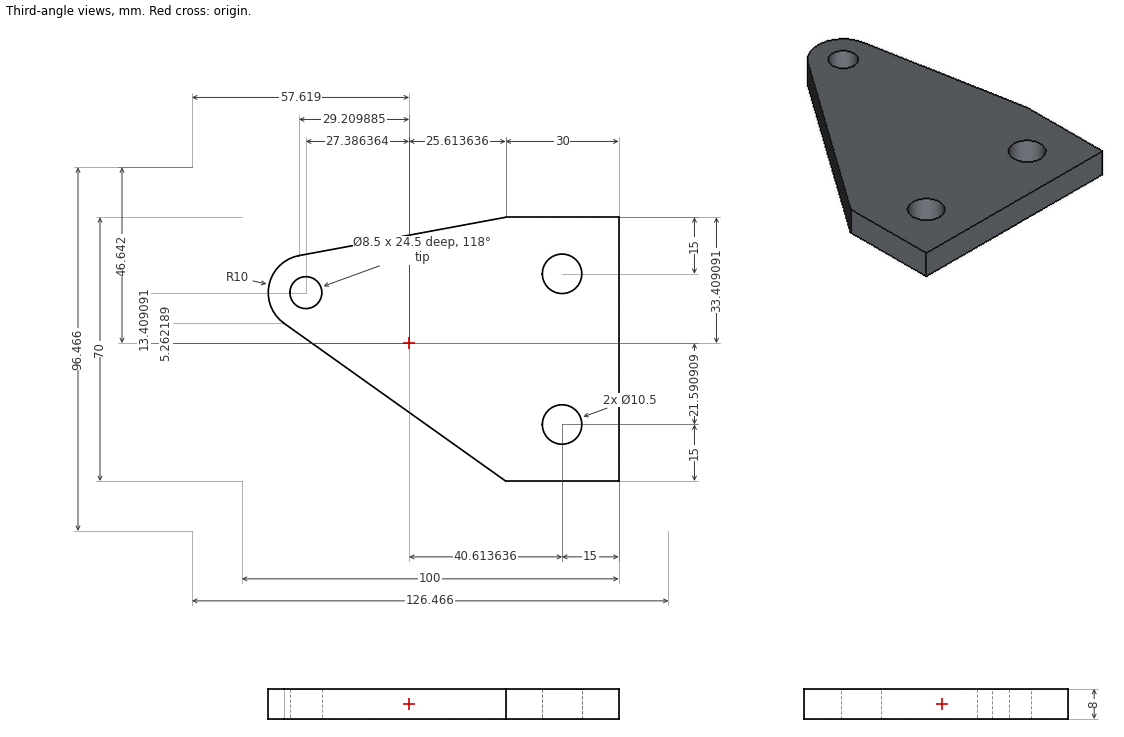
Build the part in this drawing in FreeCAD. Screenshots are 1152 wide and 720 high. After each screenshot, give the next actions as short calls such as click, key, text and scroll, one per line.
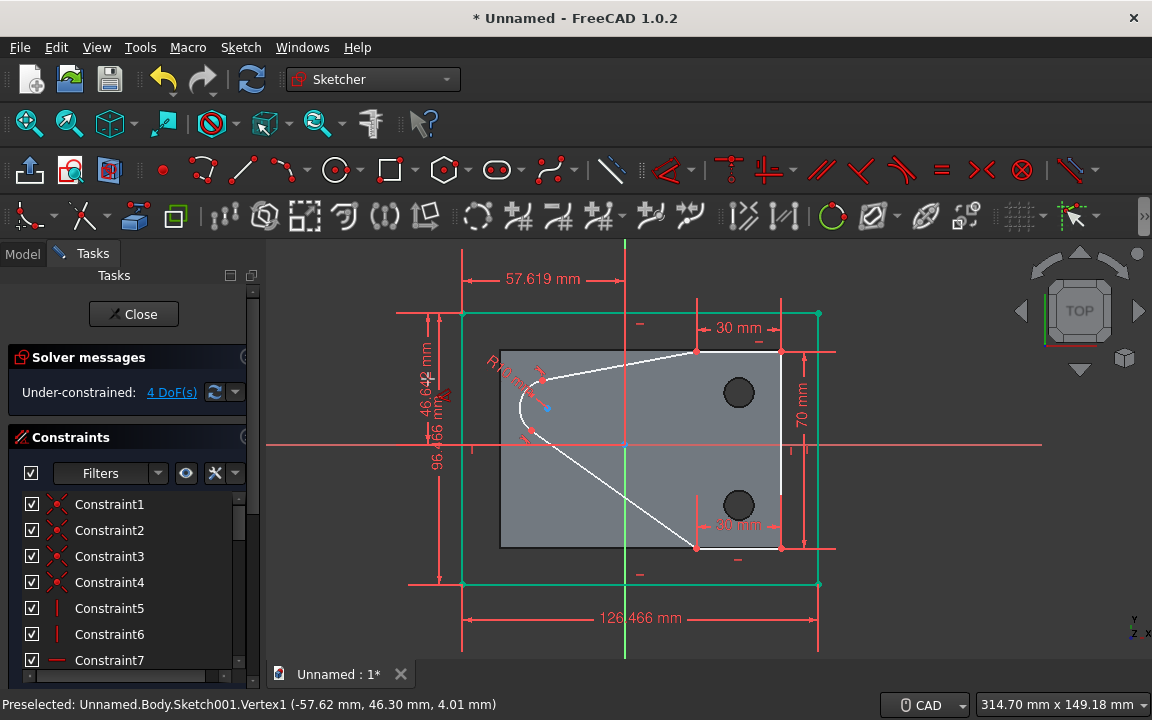
scroll(532, 431, up, 5)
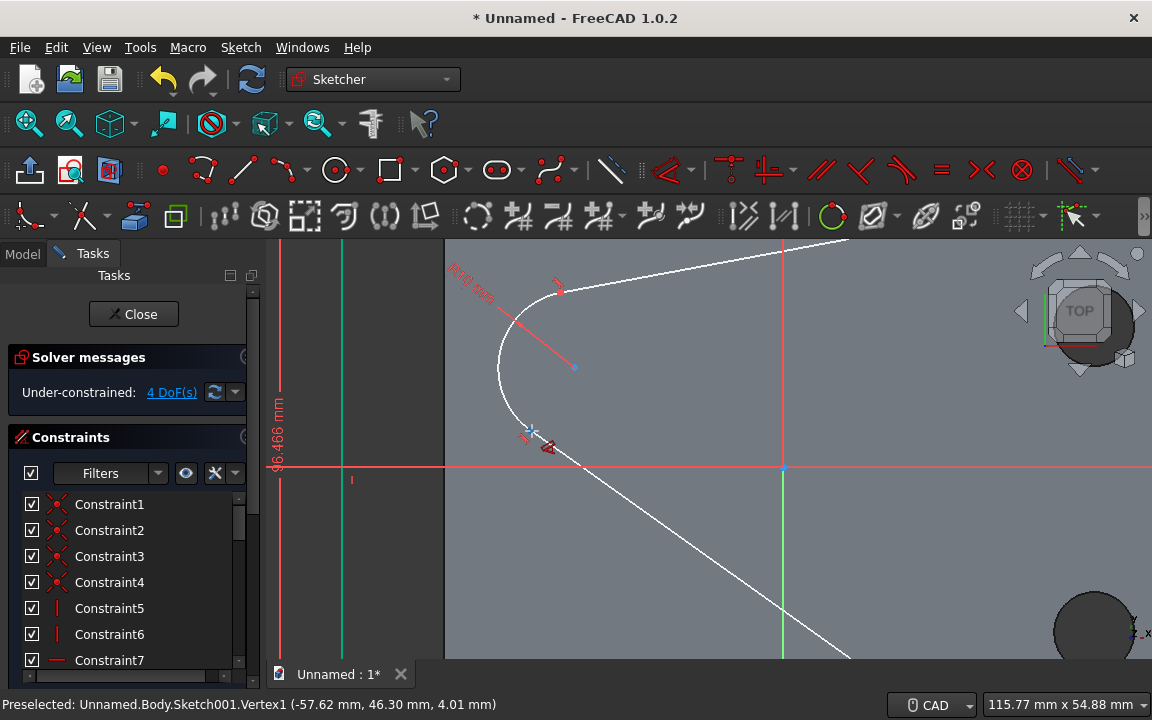
click(530, 430)
click(496, 449)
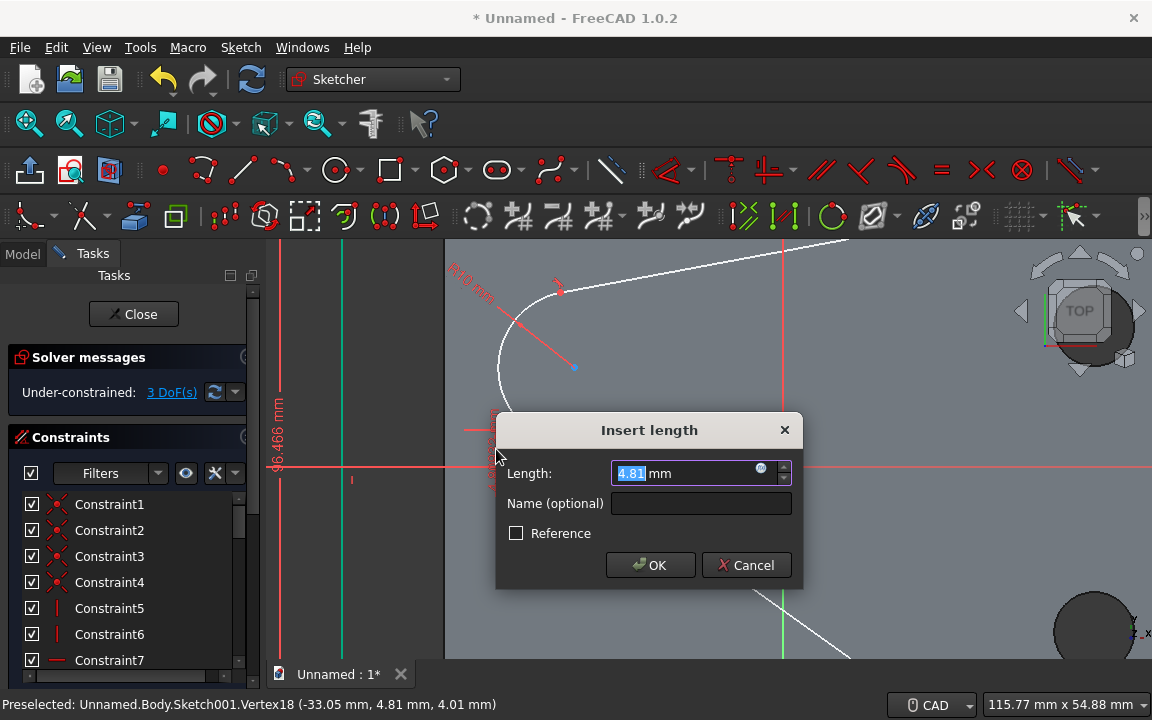
text(5.262189)
key(Return)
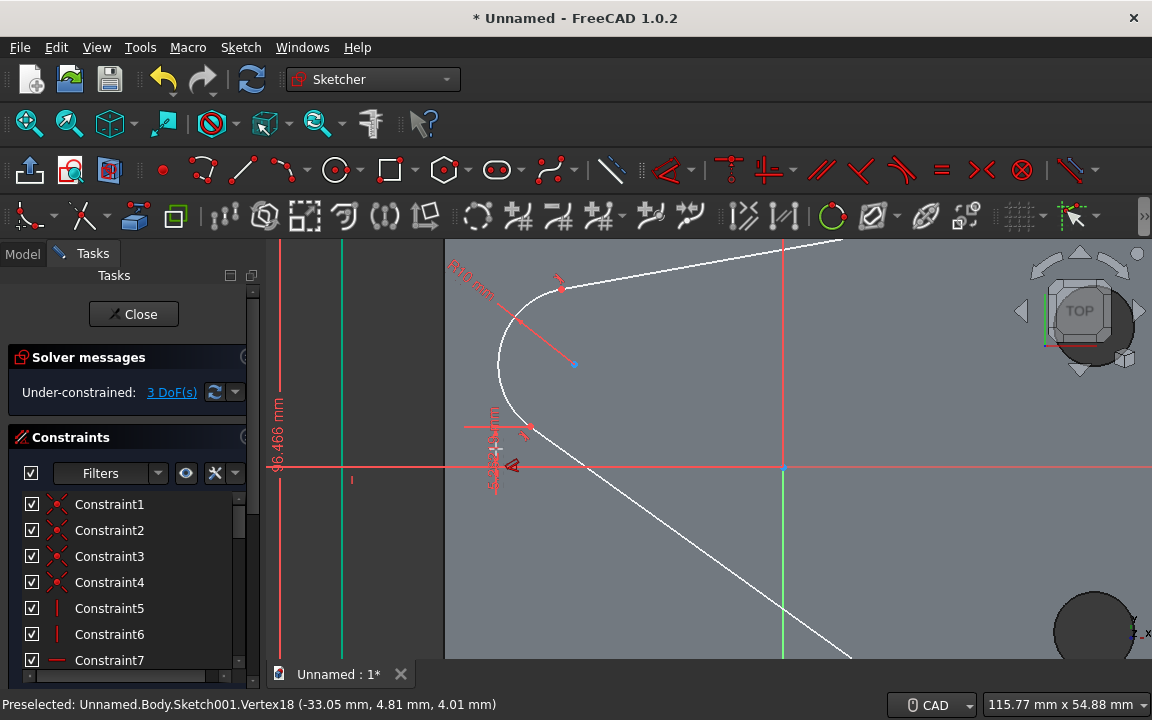
click(561, 289)
click(672, 501)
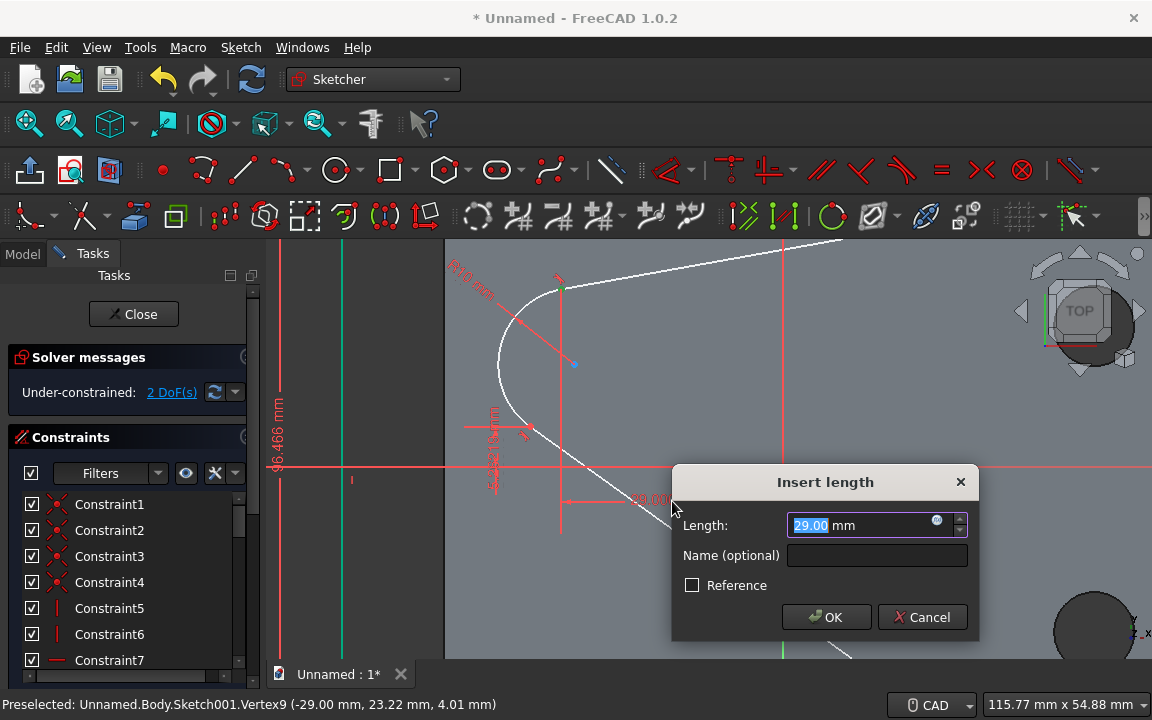
text(29.209885)
key(Return)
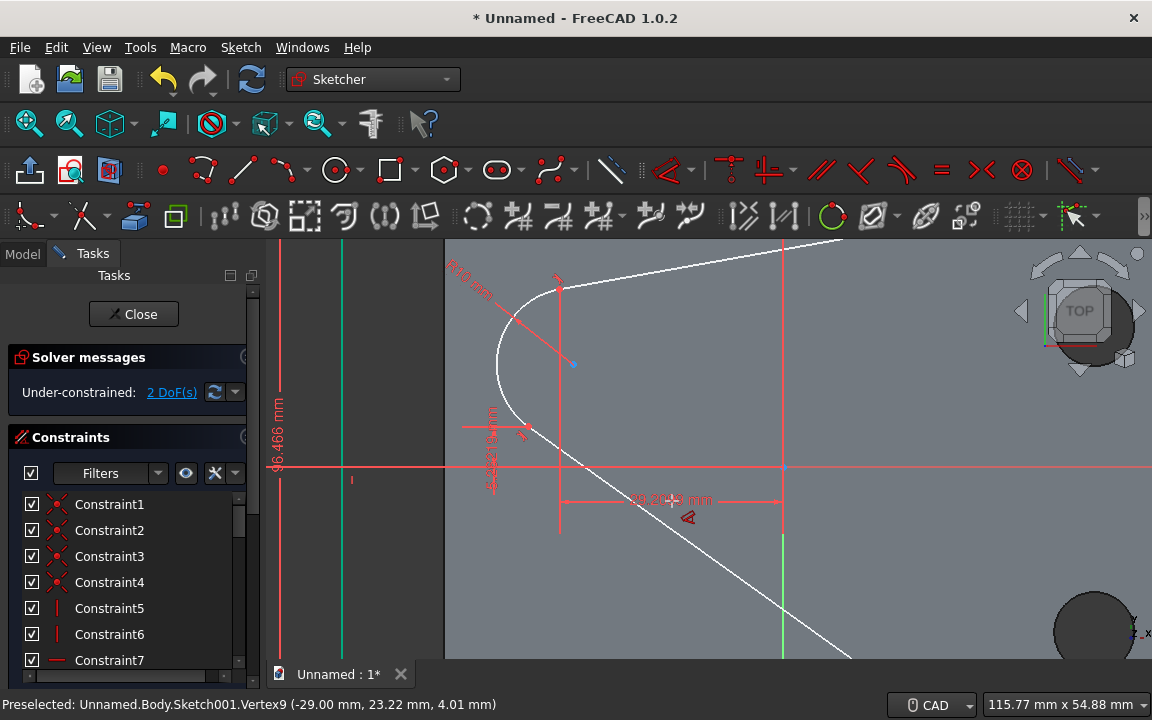
scroll(532, 431, down, 5)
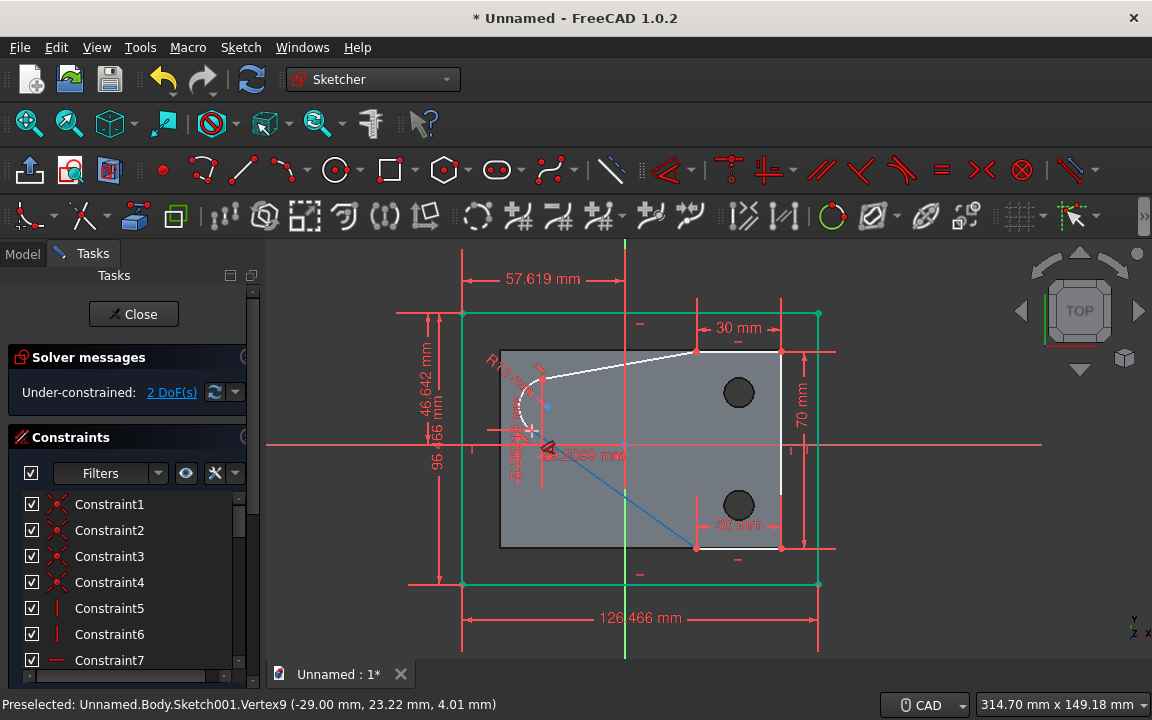
click(697, 352)
click(661, 479)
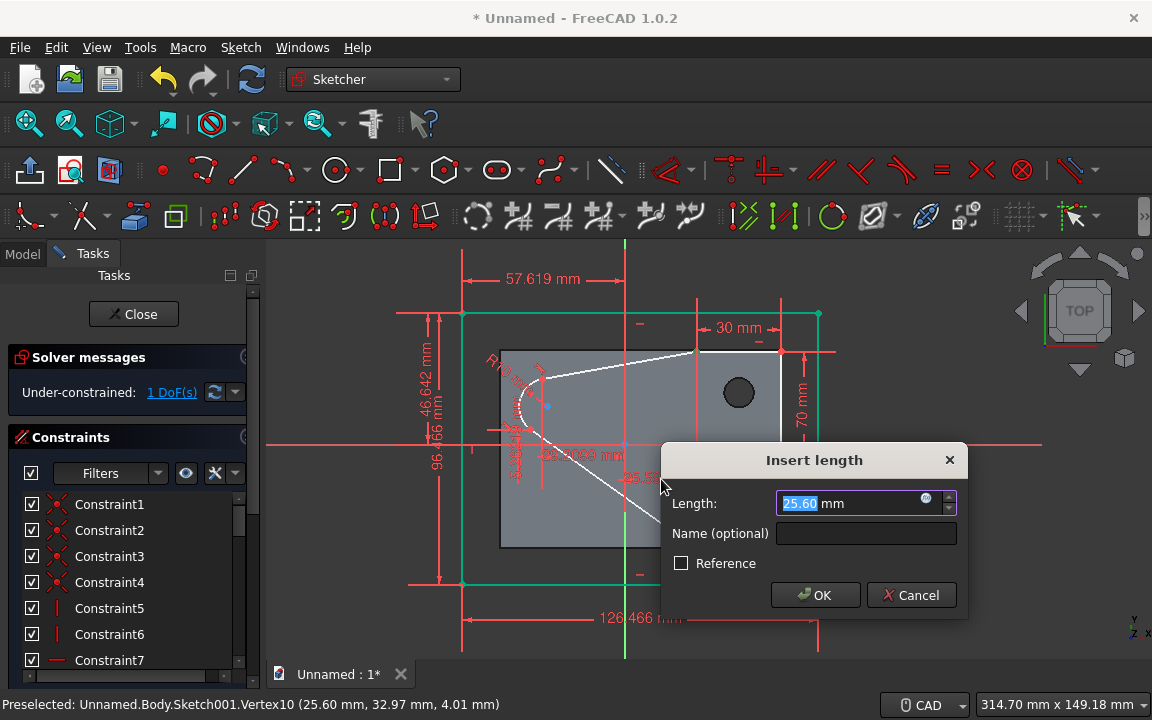
text(25.613636)
key(Return)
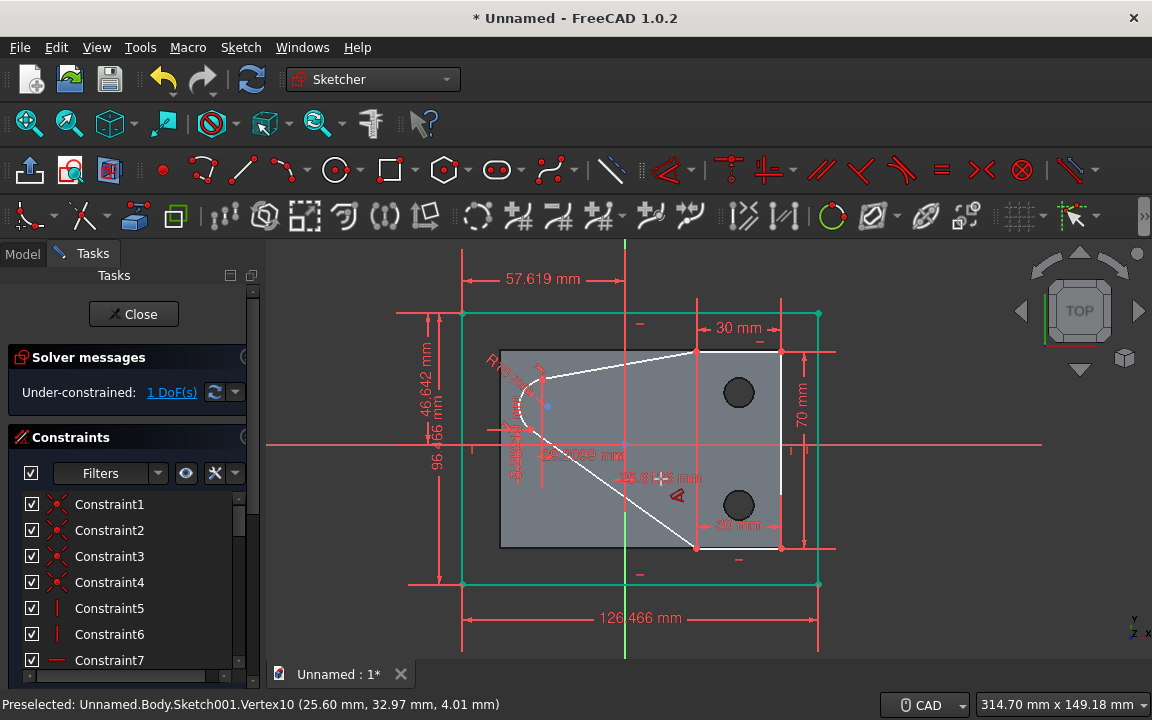
click(697, 352)
click(731, 398)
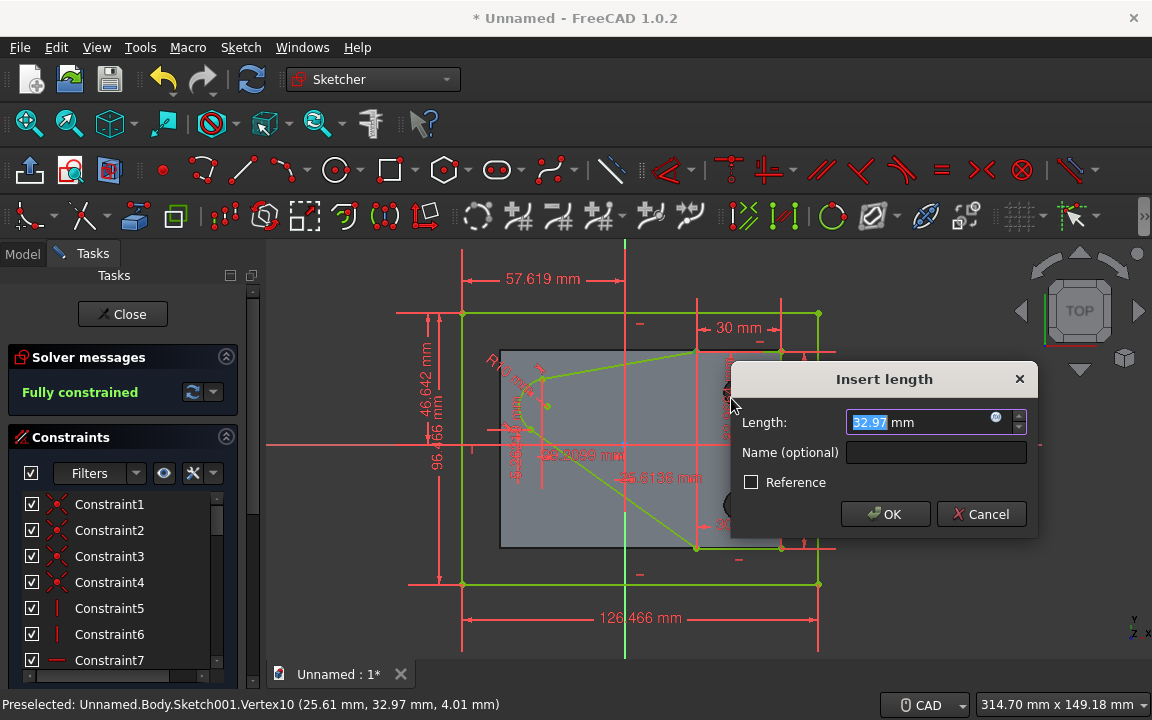
text(33.409091)
key(Return)
key(Escape)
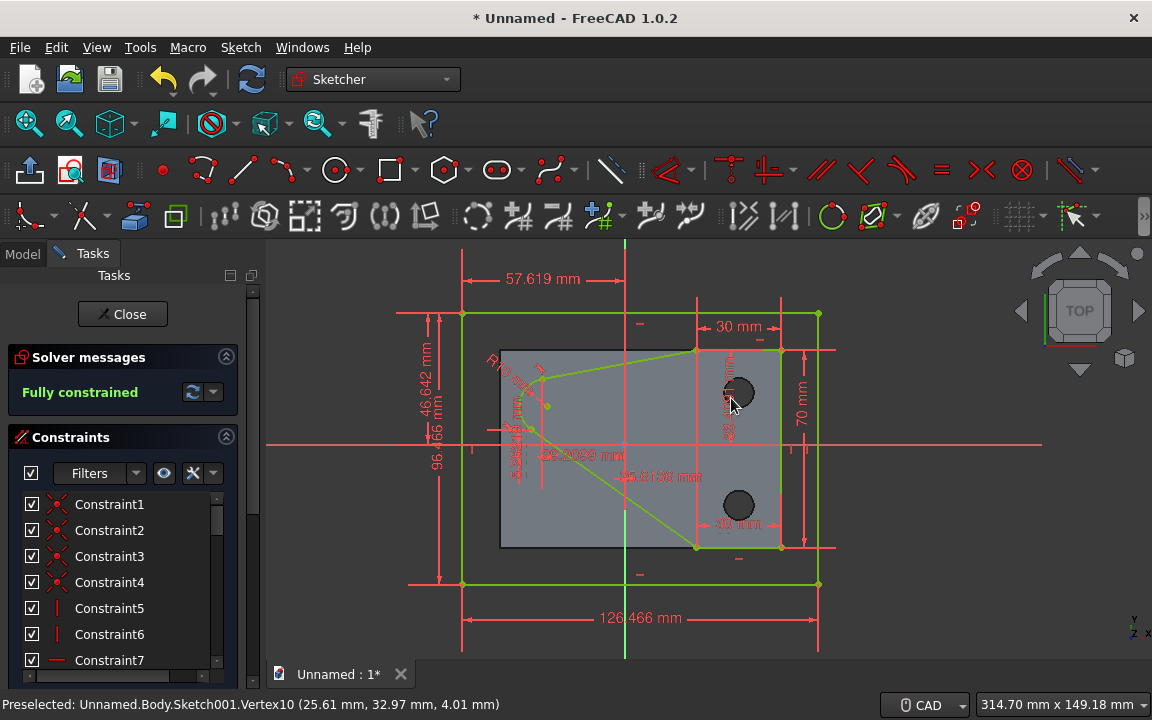
click(123, 314)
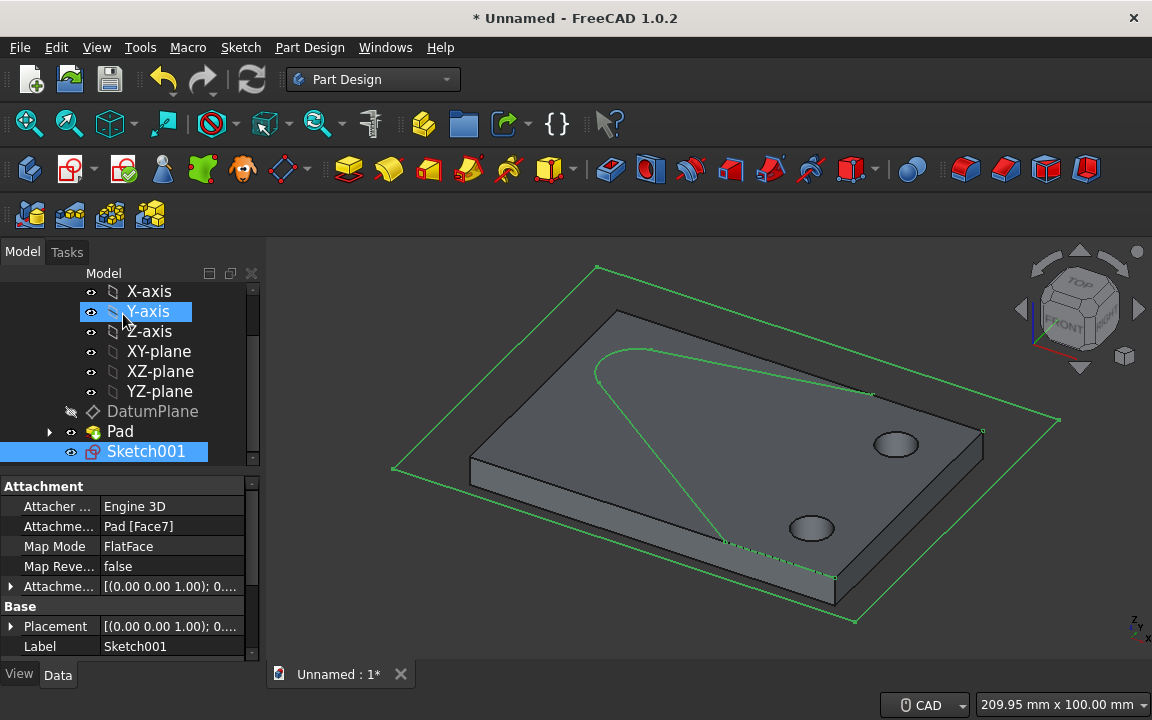
click(612, 170)